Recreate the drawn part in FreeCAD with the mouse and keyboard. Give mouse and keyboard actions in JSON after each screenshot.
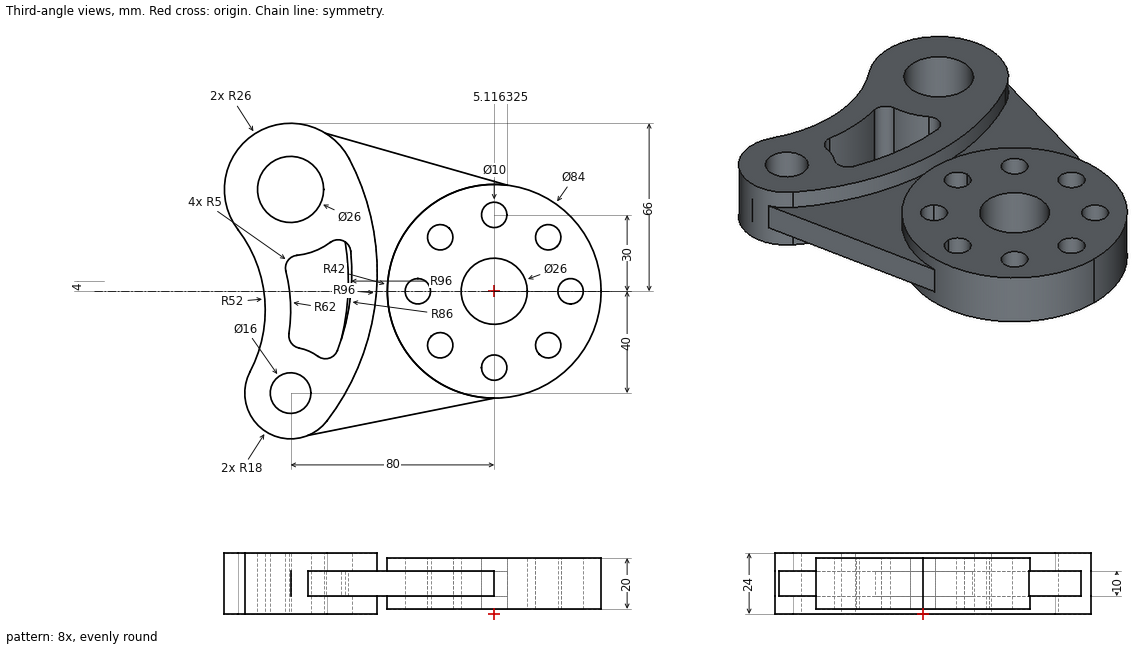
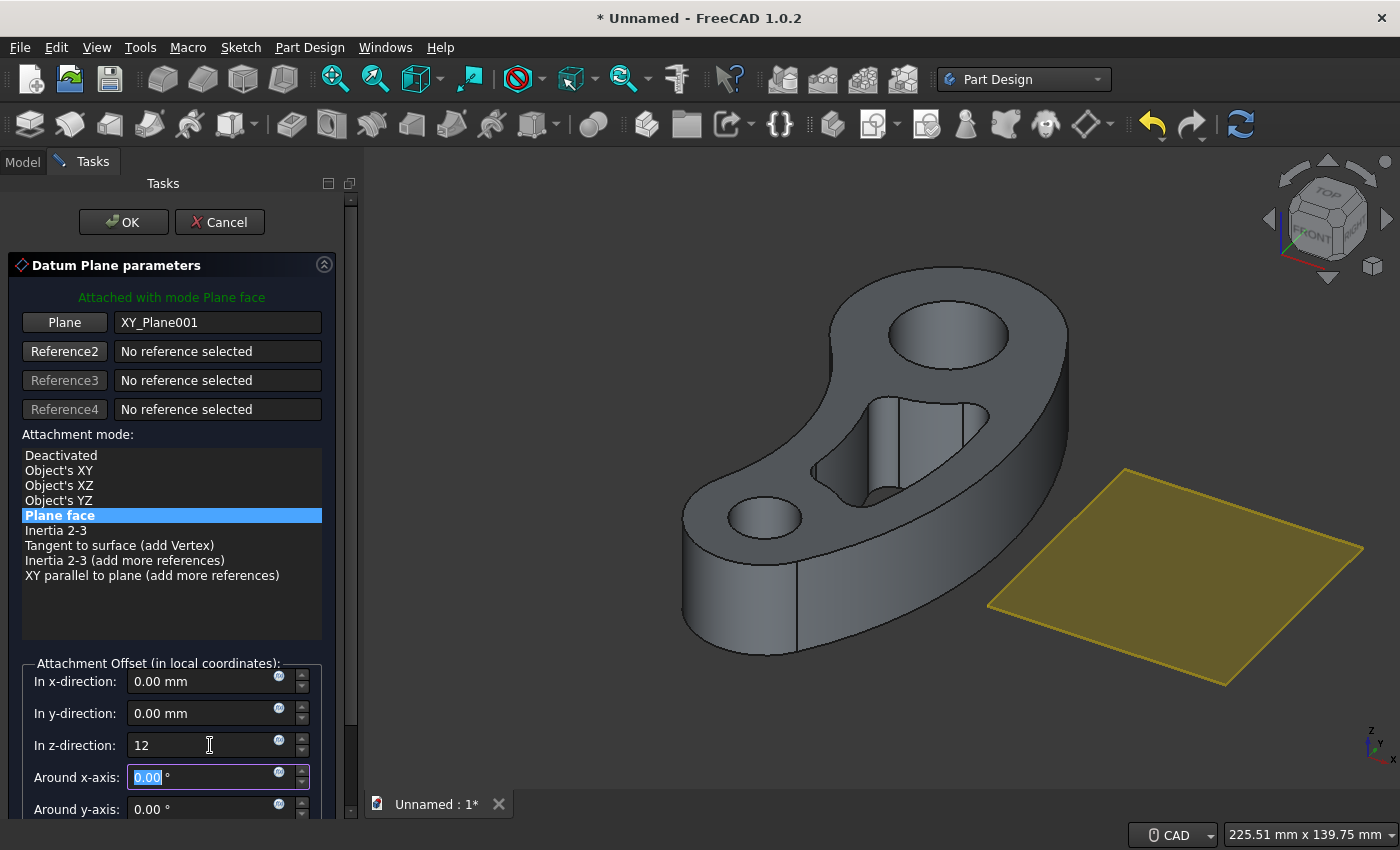
{"action": "left_click", "coordinate": [124, 222]}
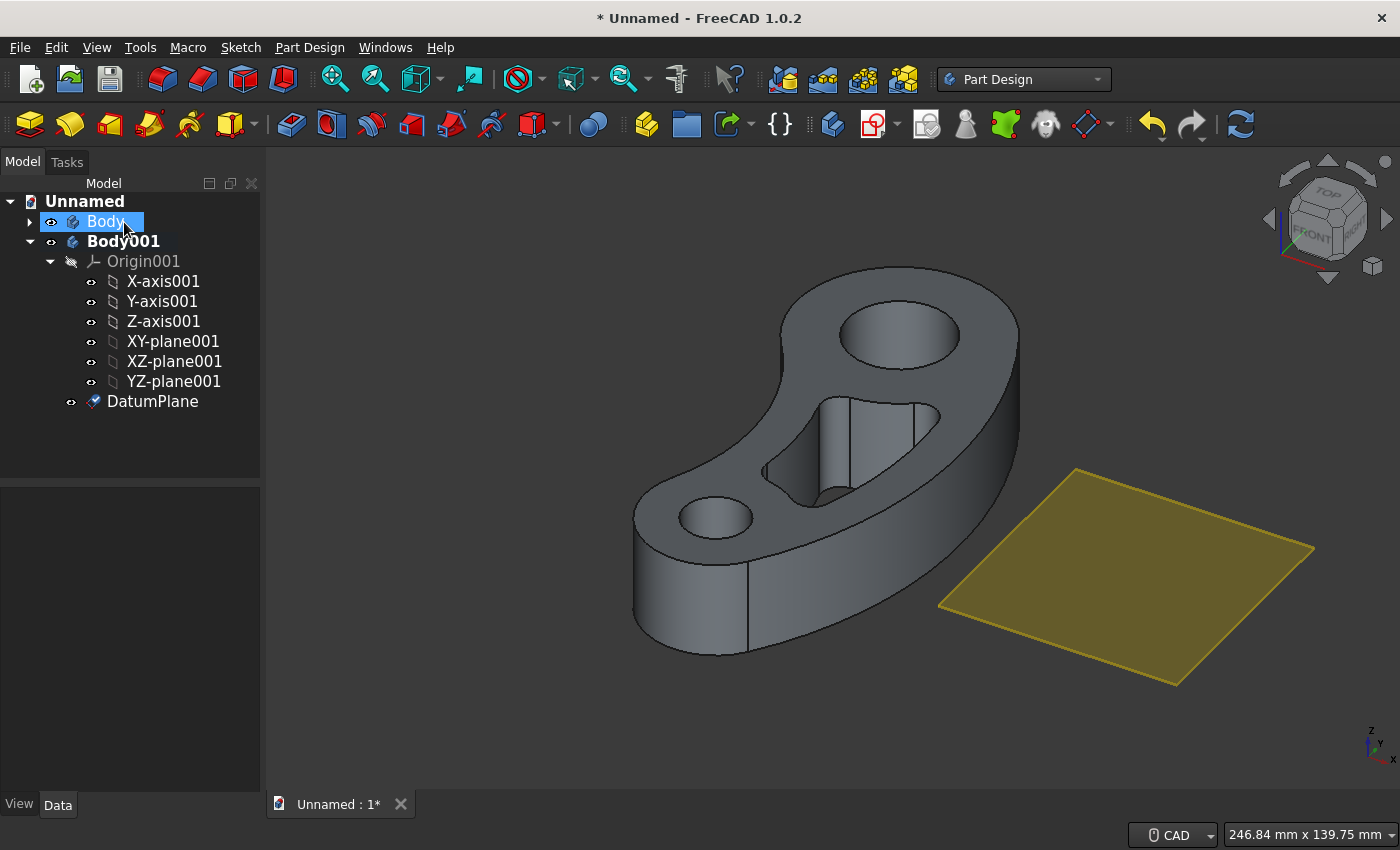
{"action": "left_click", "coordinate": [116, 402]}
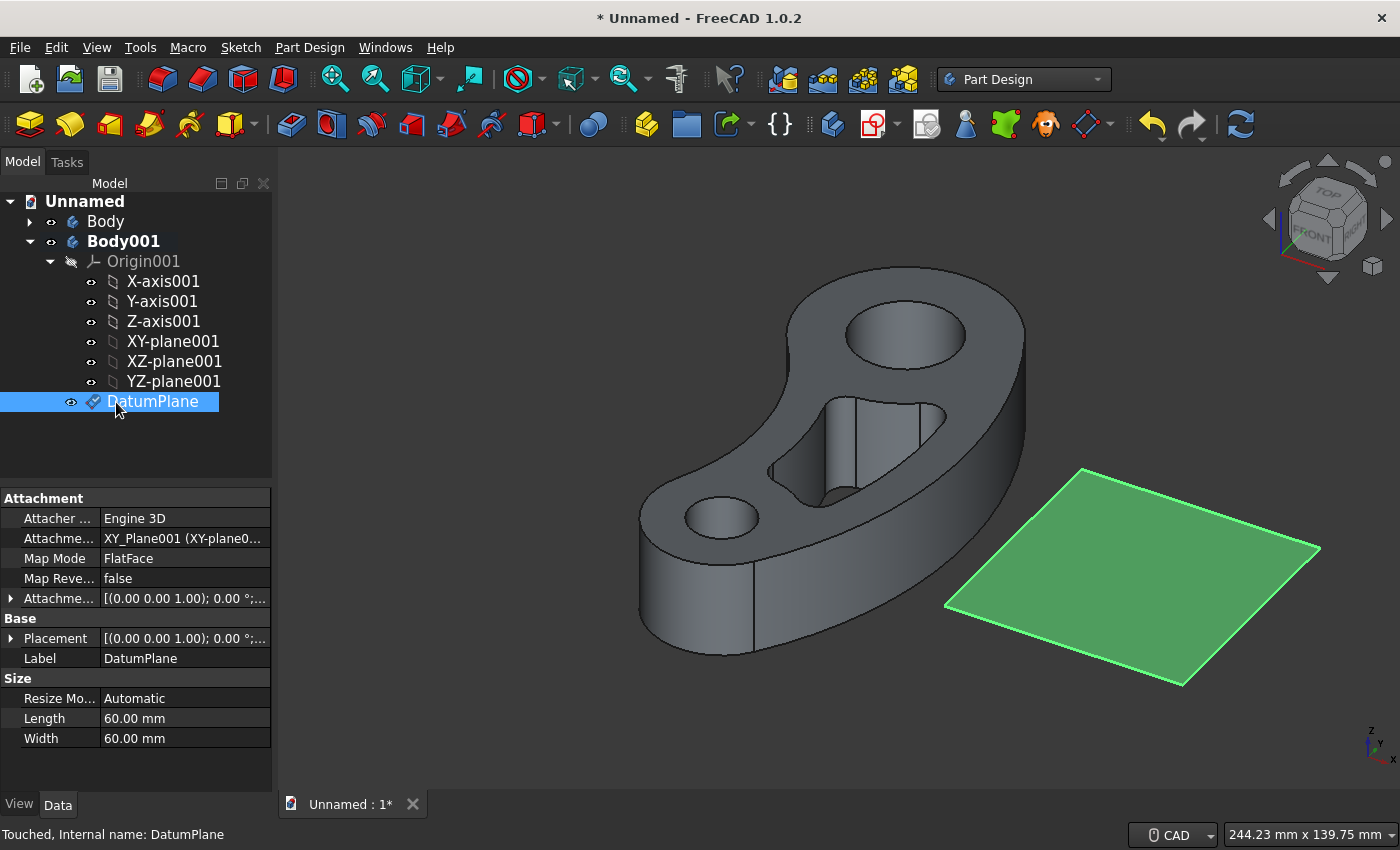
{"action": "left_click", "coordinate": [874, 124]}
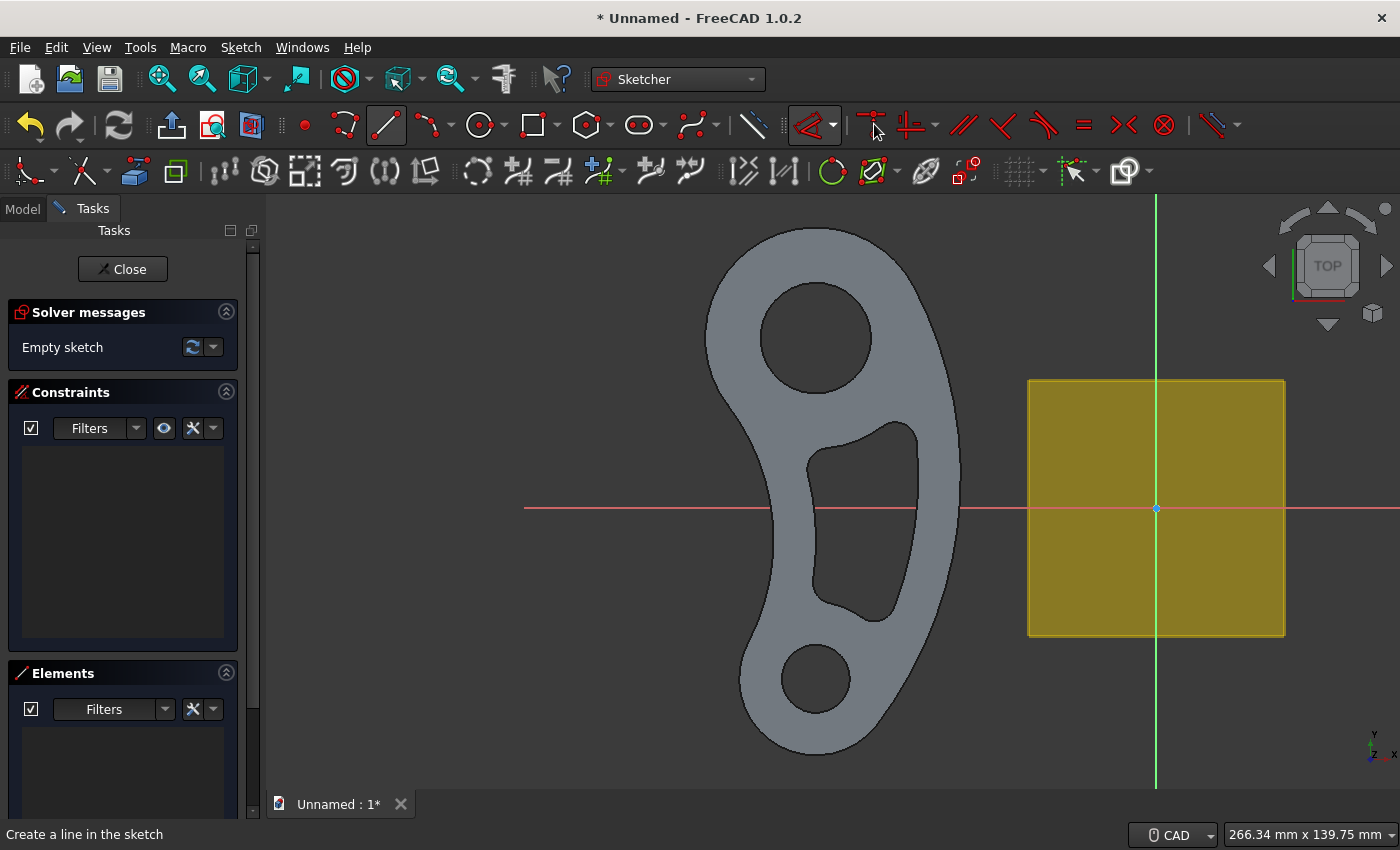
{"action": "scroll", "coordinate": [294, 415], "scroll_direction": "down", "scroll_amount": 1}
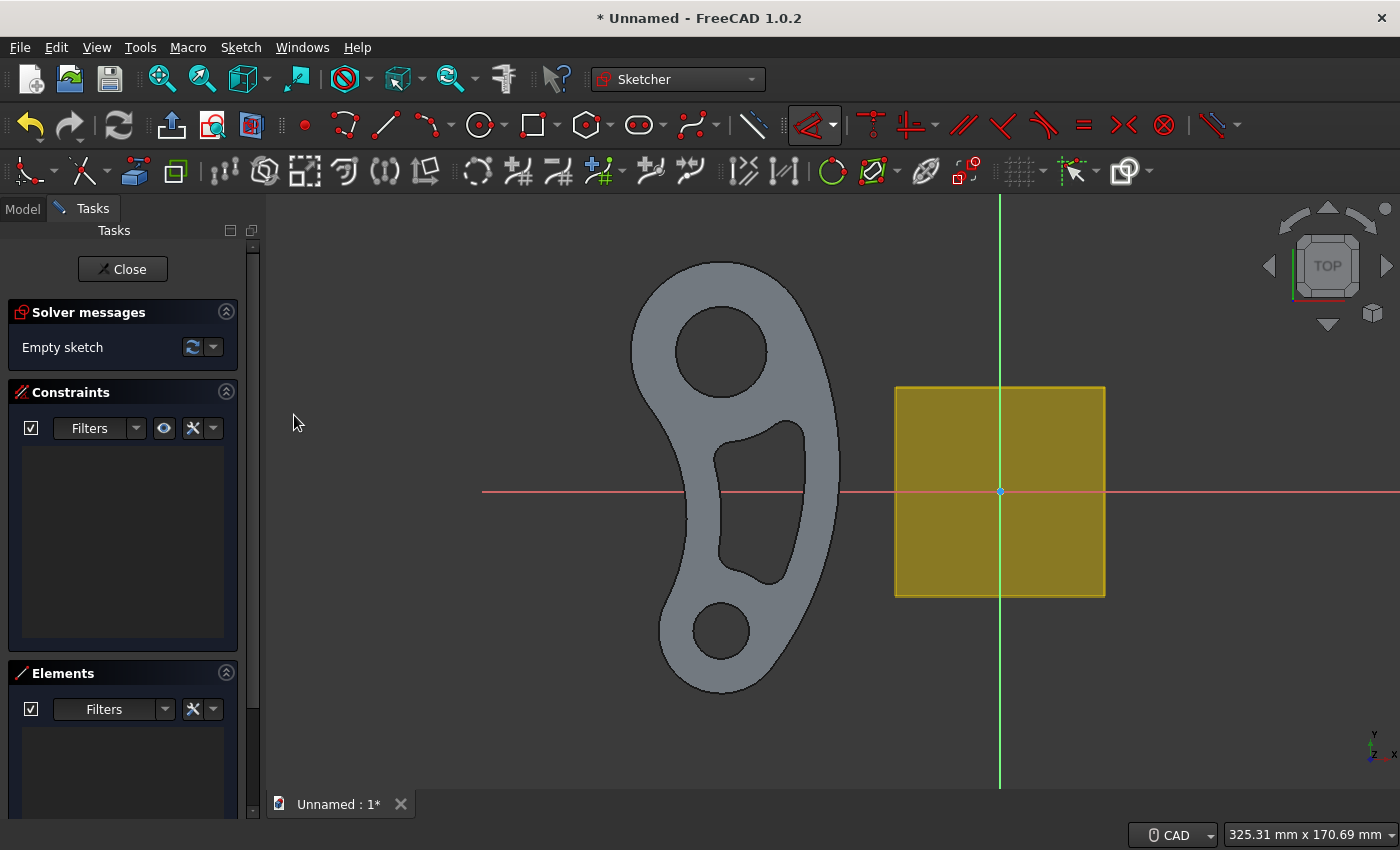
{"action": "left_click", "coordinate": [480, 126]}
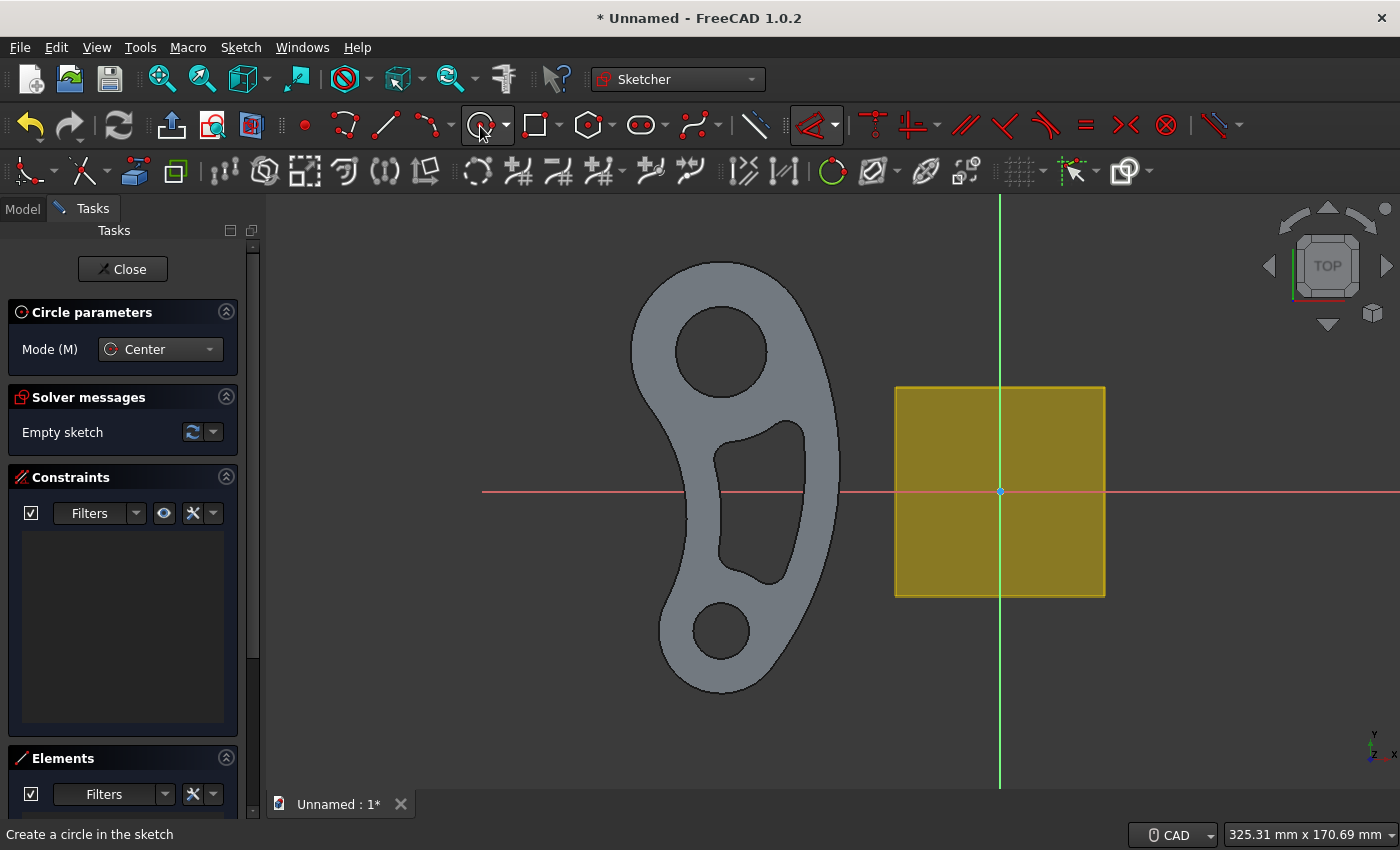
{"action": "left_click", "coordinate": [1000, 492]}
{"action": "left_click", "coordinate": [1104, 388]}
{"action": "key", "text": "Escape"}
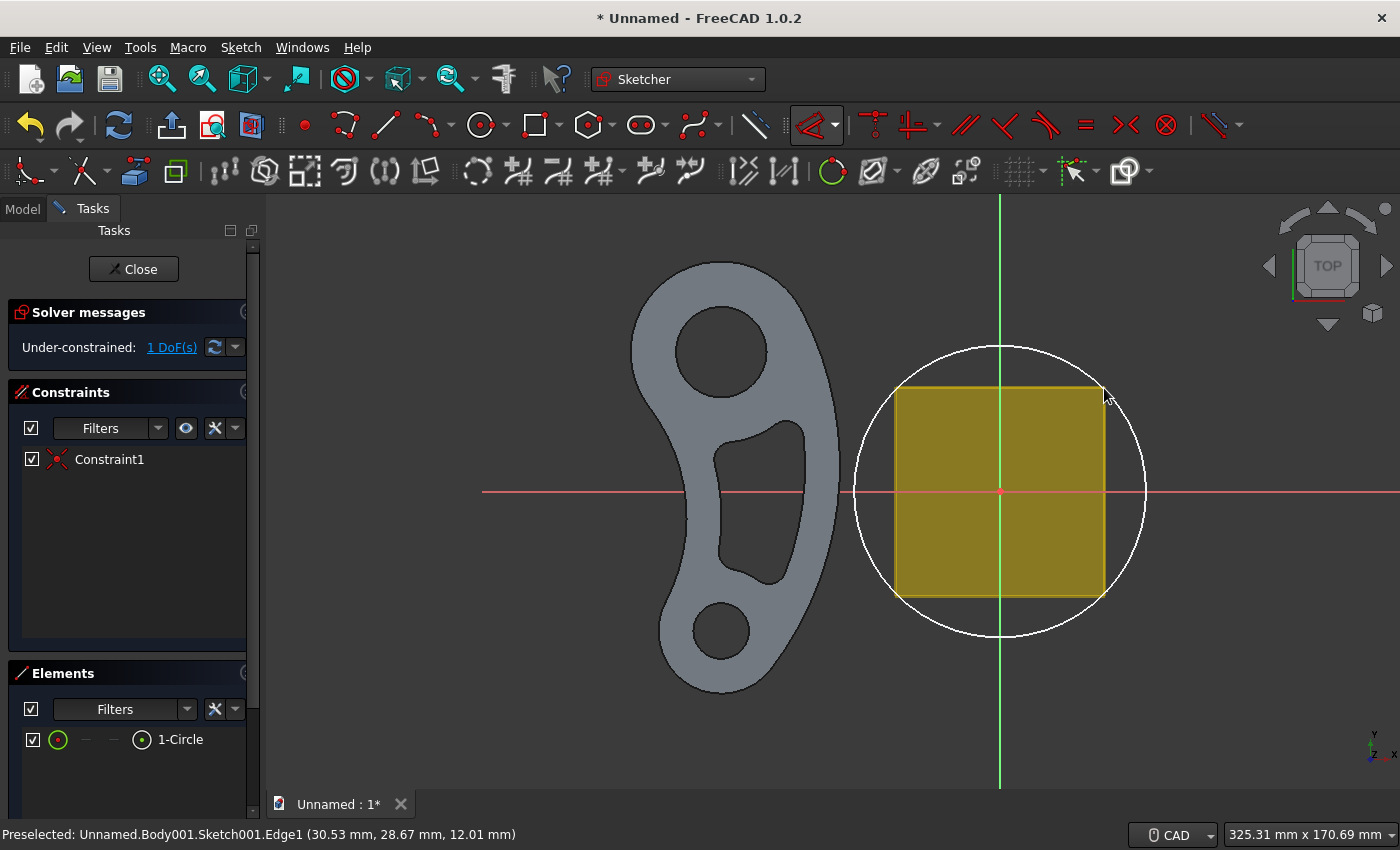
{"action": "left_click", "coordinate": [1103, 388]}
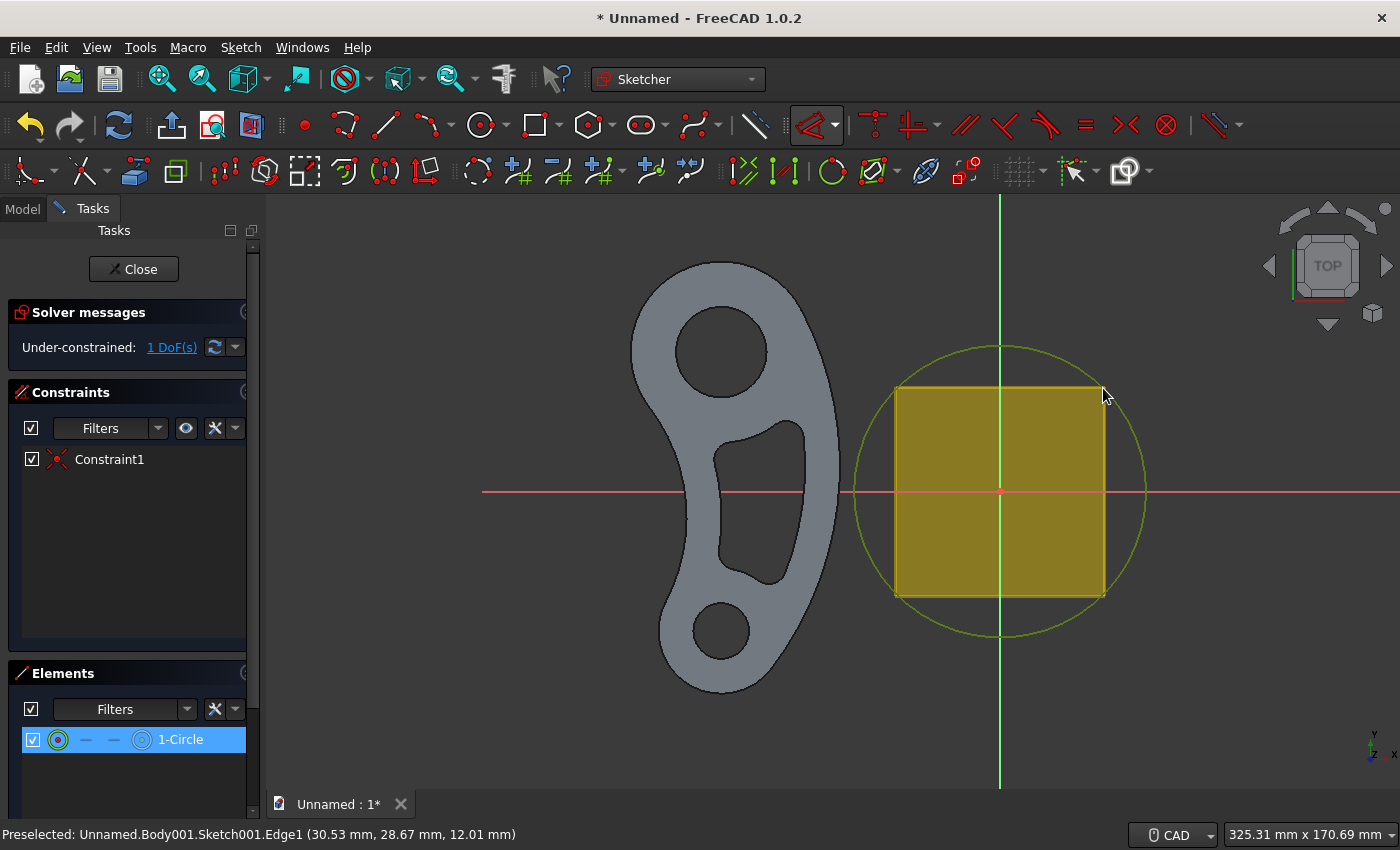
{"action": "left_click", "coordinate": [838, 126]}